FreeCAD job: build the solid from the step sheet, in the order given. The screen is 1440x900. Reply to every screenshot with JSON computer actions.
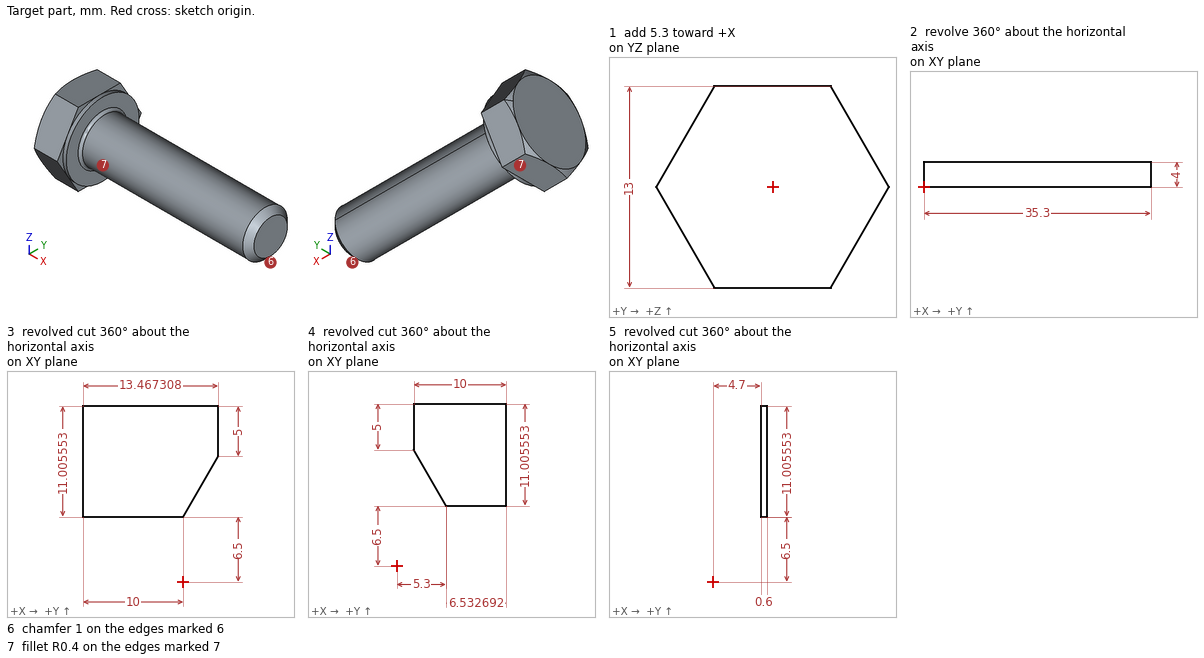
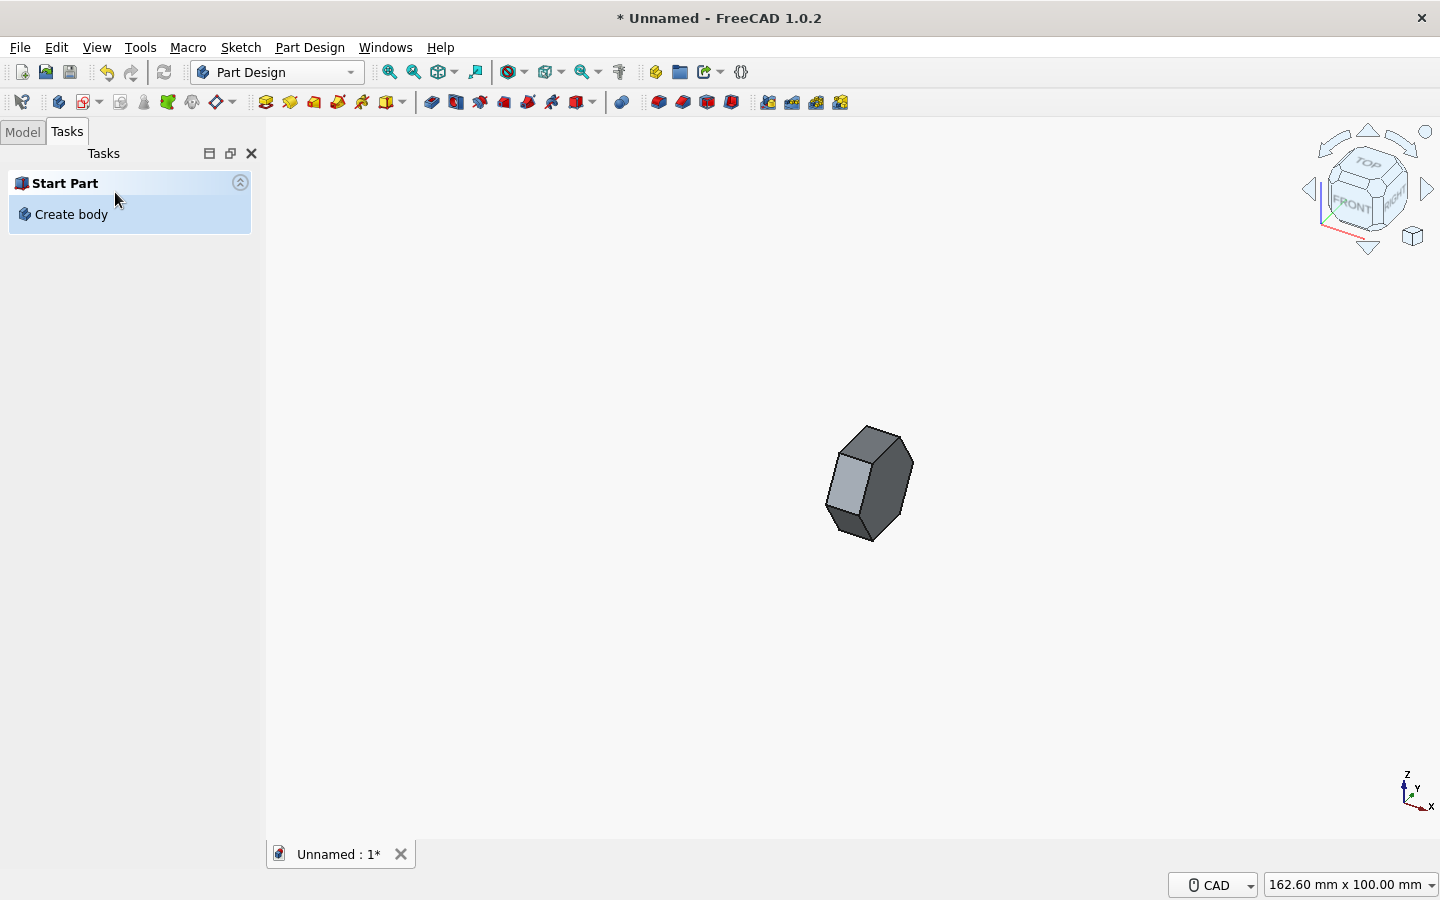
{"action": "key", "text": "v f"}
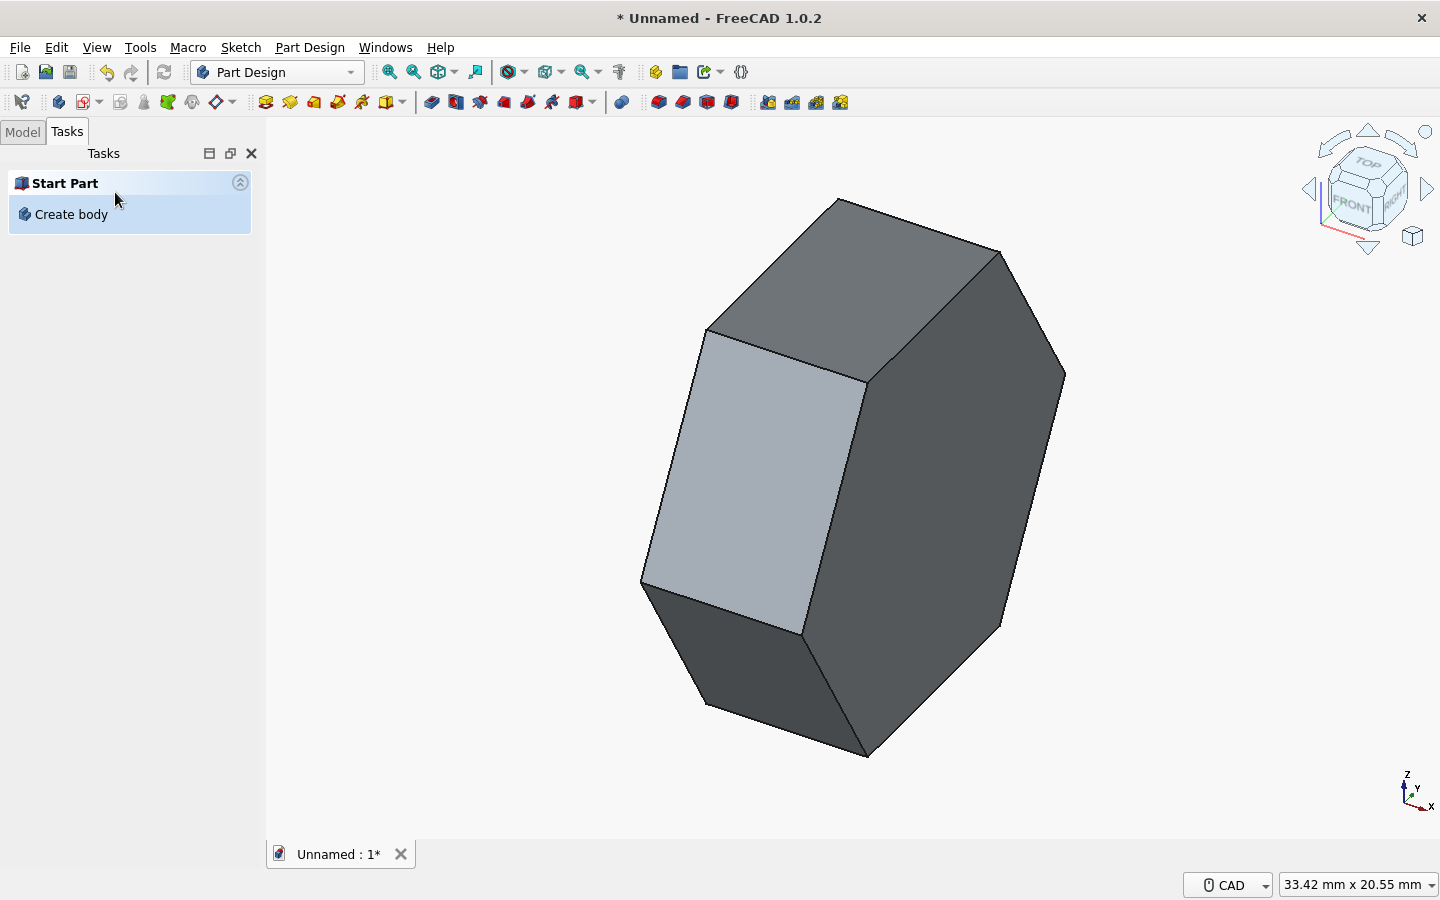
{"action": "left_click", "coordinate": [84, 102]}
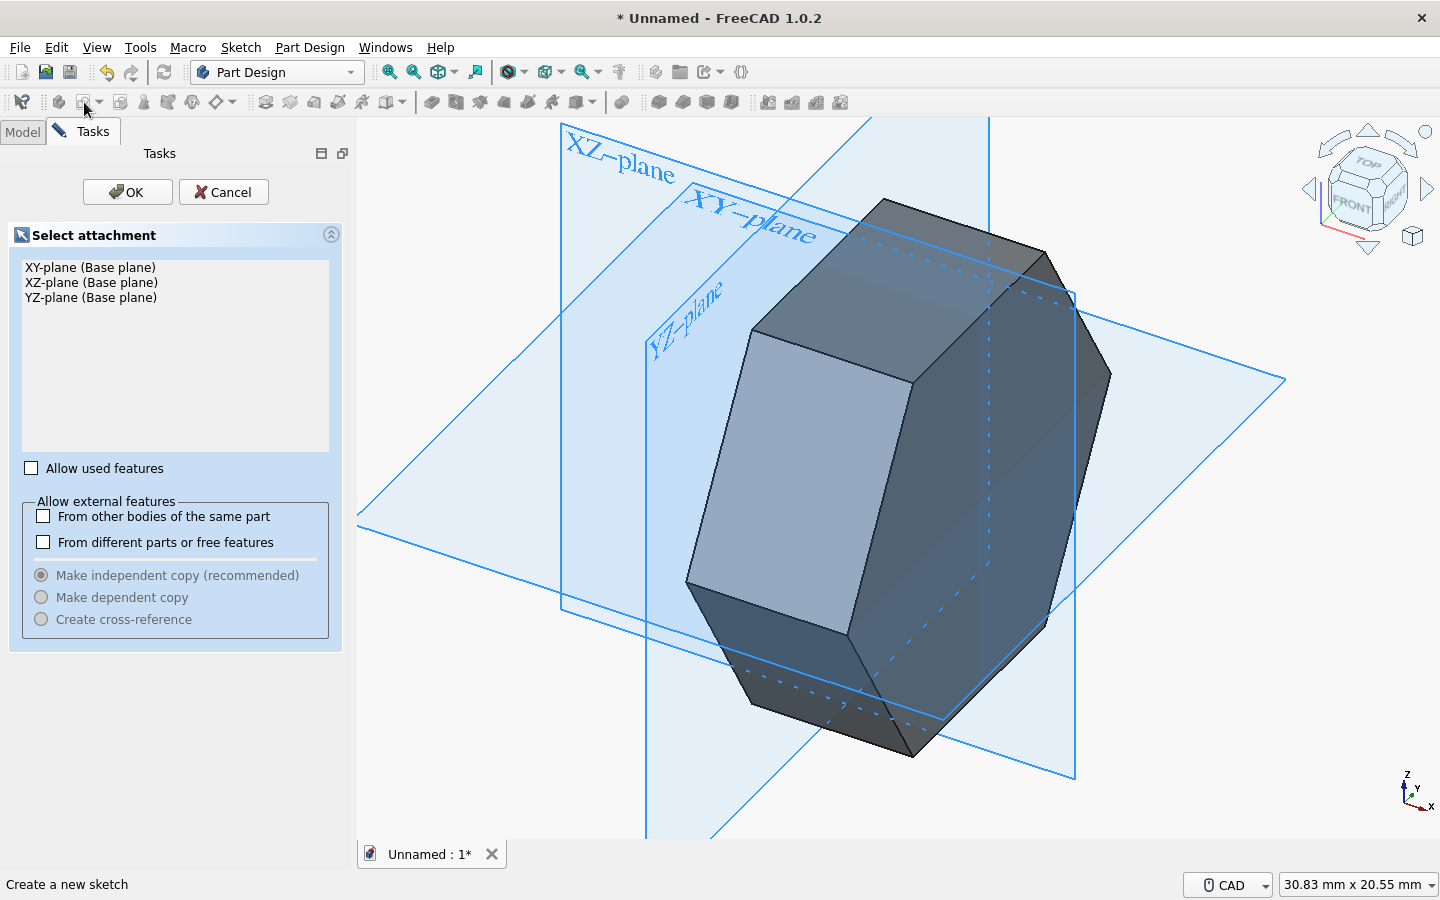
{"action": "left_click", "coordinate": [82, 268]}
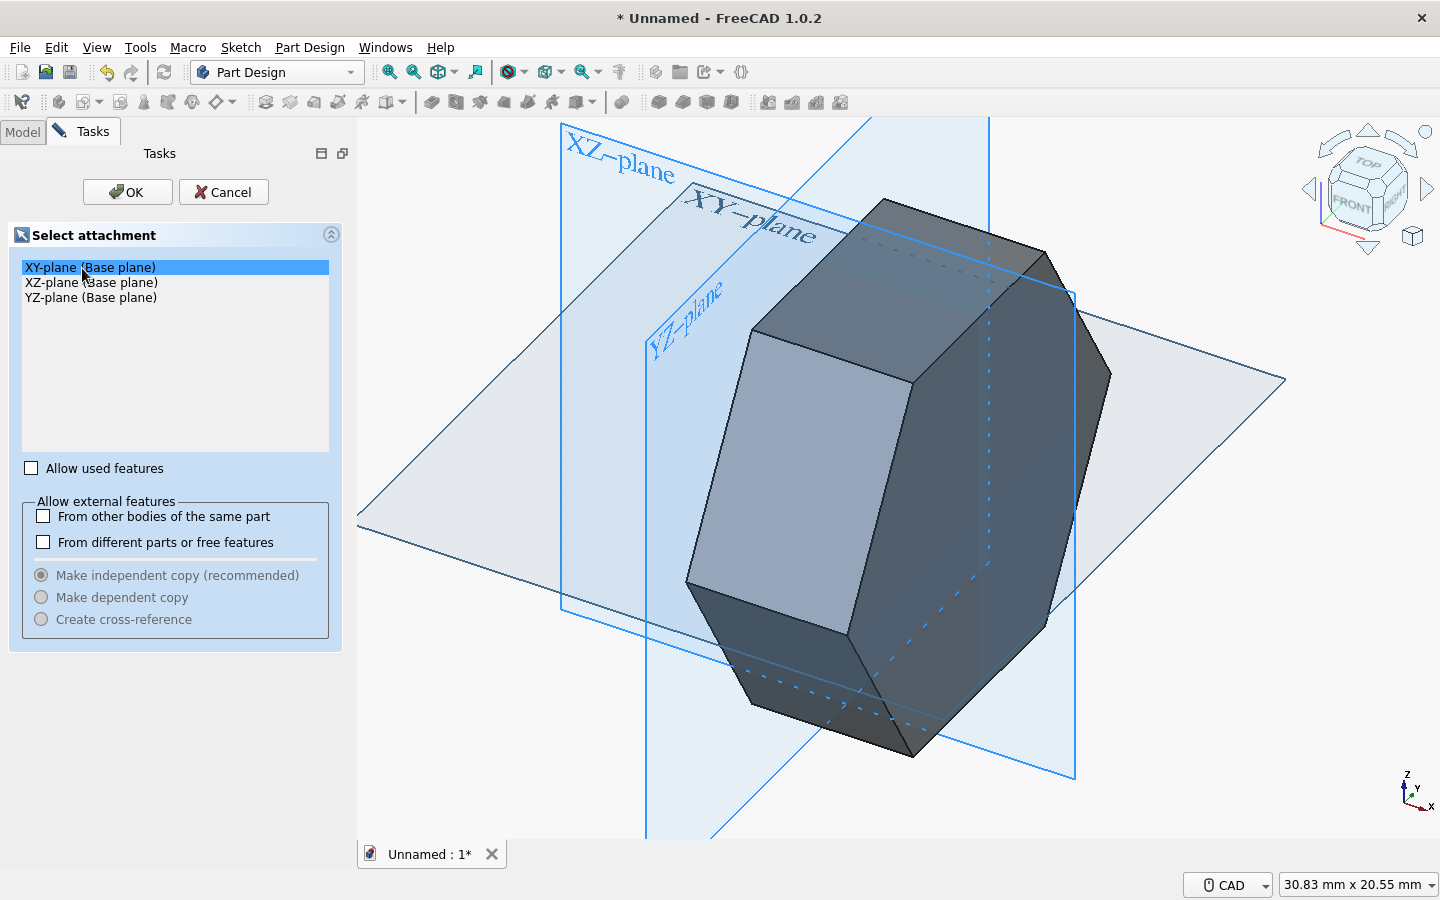
{"action": "left_click", "coordinate": [128, 192]}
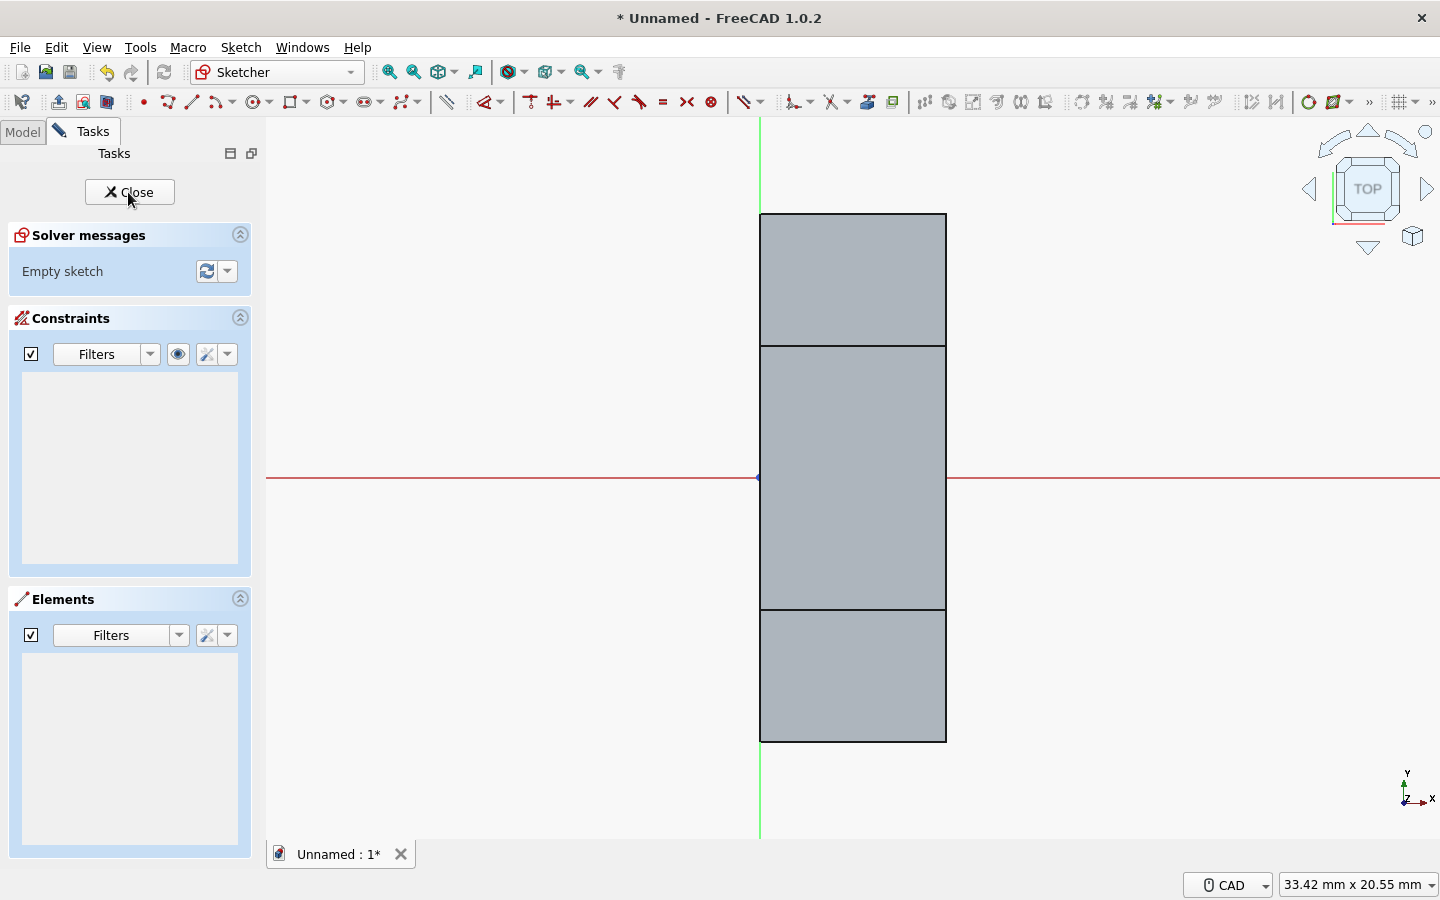
{"action": "key", "text": "q s"}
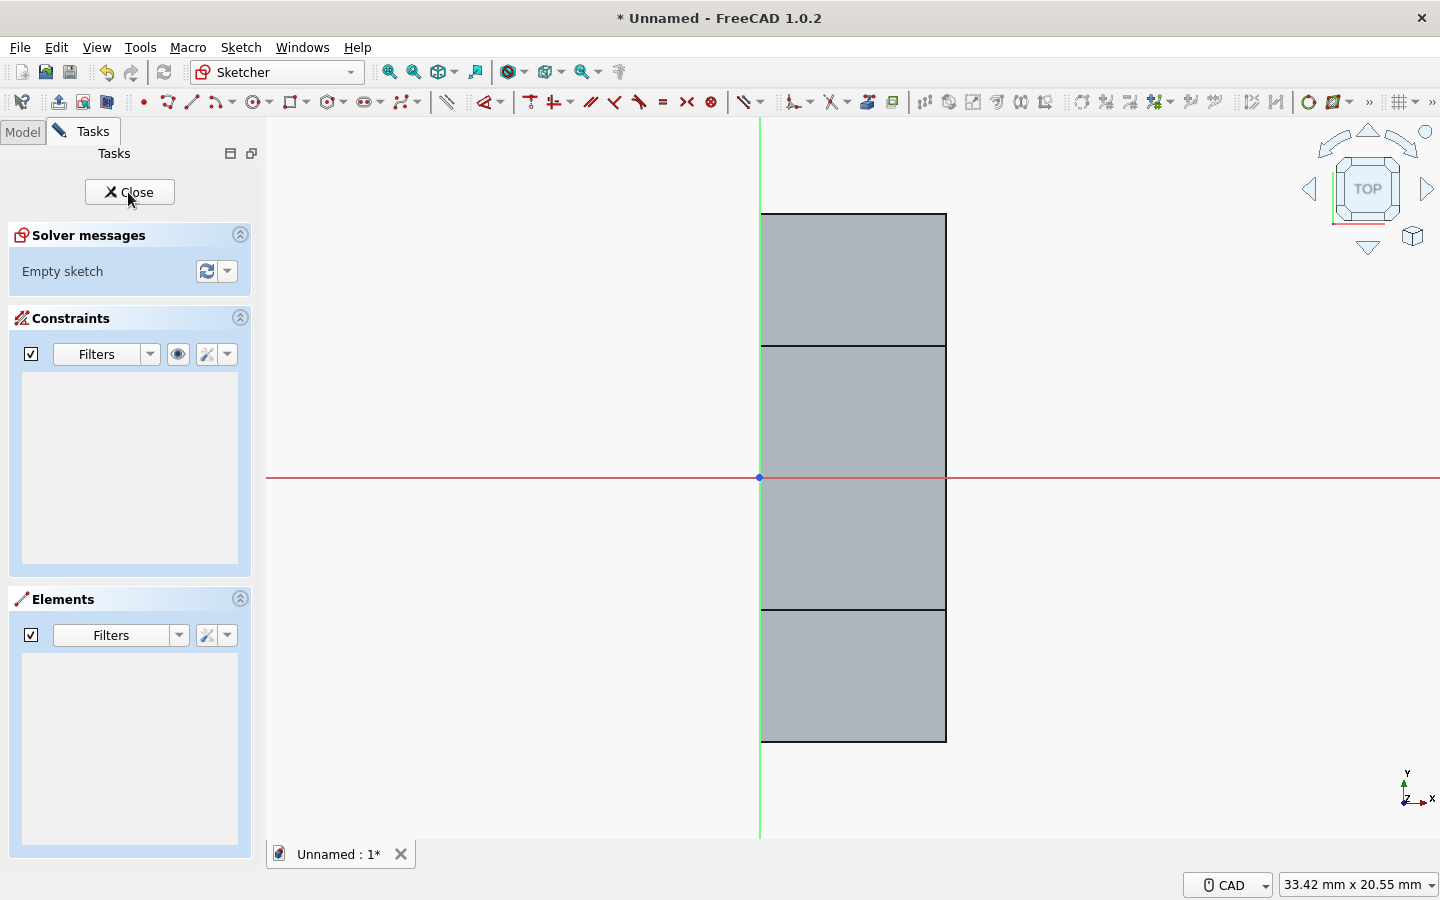
{"action": "scroll", "coordinate": [294, 563], "scroll_direction": "down", "scroll_amount": 3}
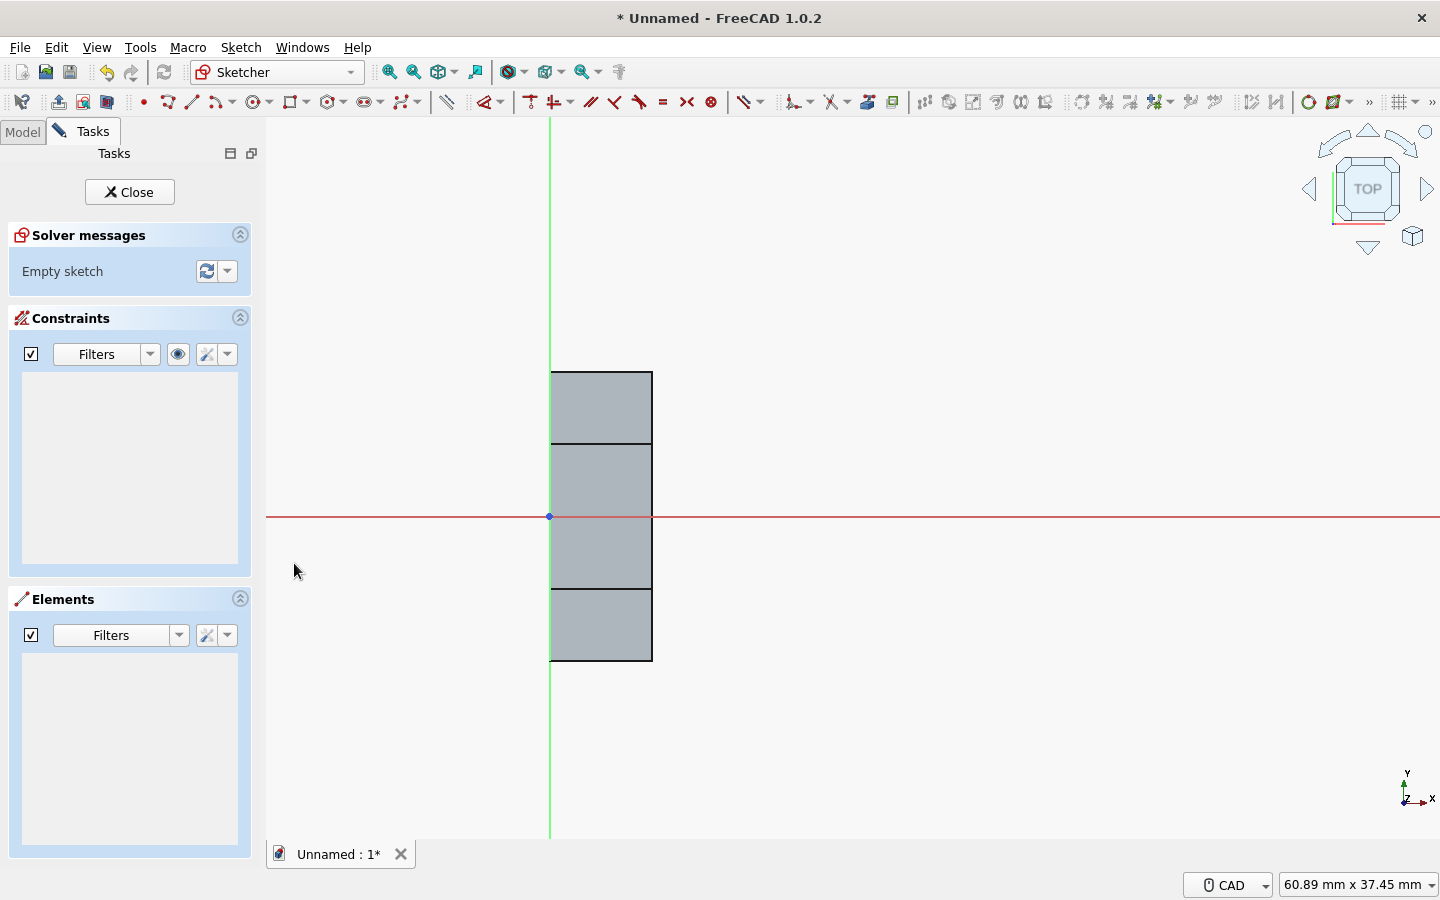
{"action": "key", "text": "g r"}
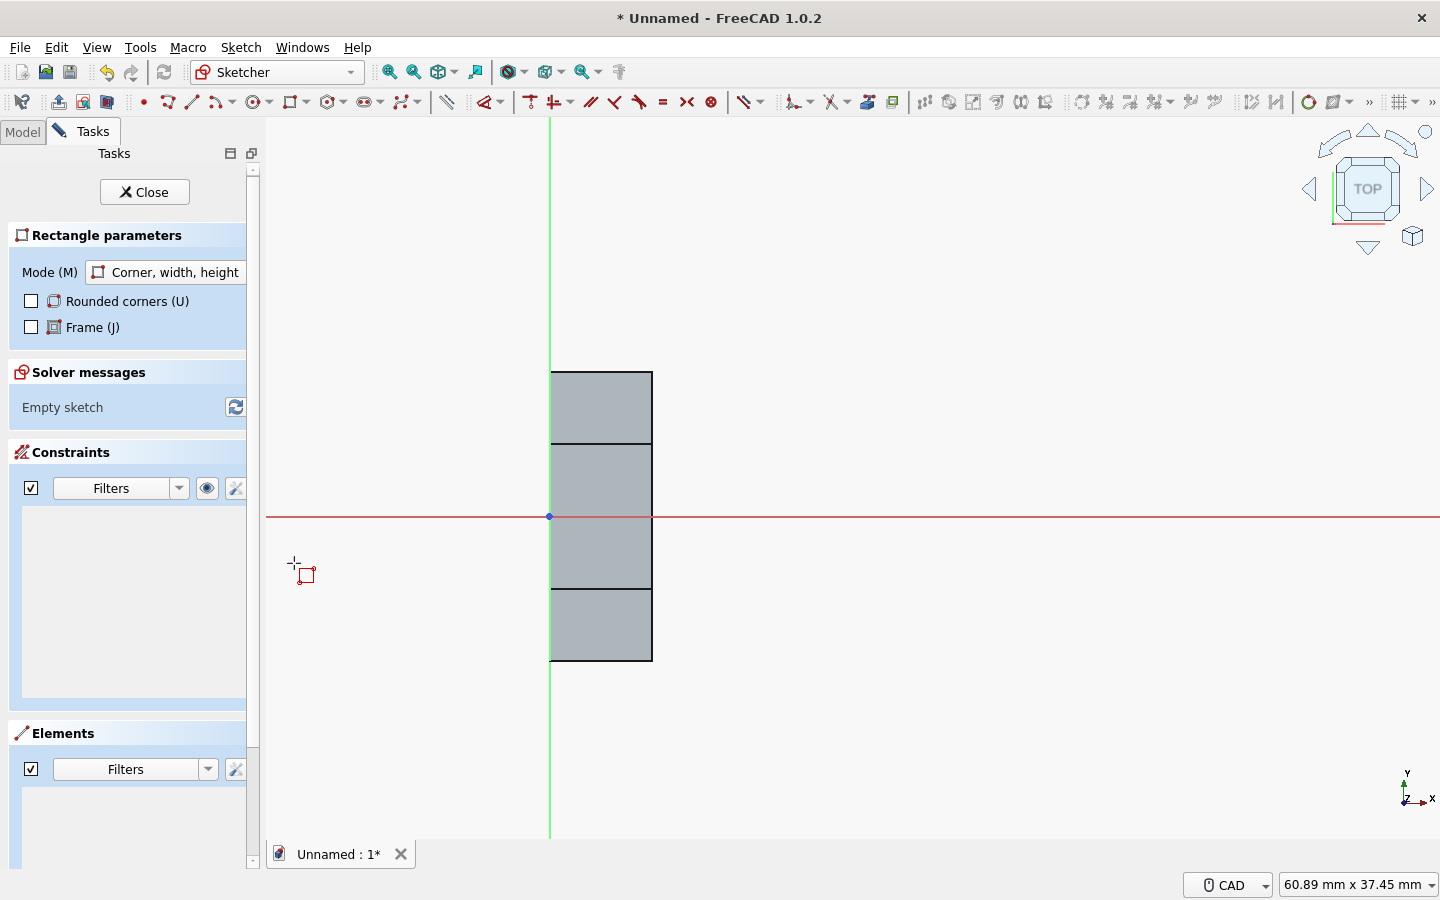
{"action": "left_click", "coordinate": [550, 517]}
{"action": "mouse_move", "coordinate": [1230, 440]}